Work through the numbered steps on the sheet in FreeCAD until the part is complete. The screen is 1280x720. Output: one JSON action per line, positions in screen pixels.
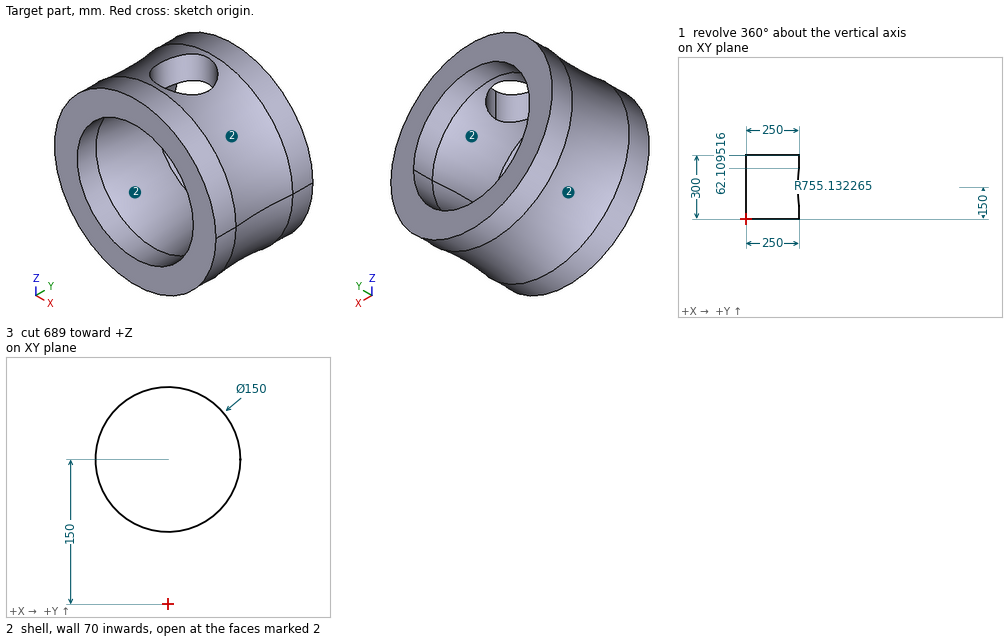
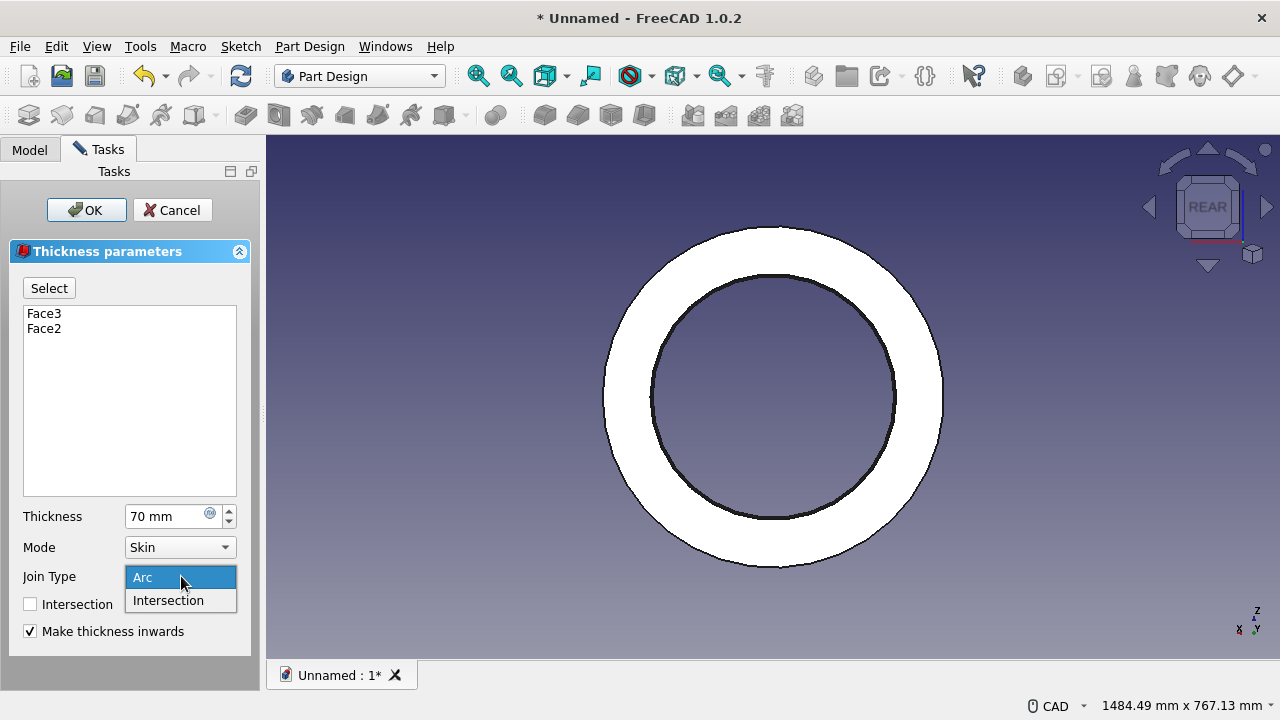
{"action": "left_click", "coordinate": [179, 600]}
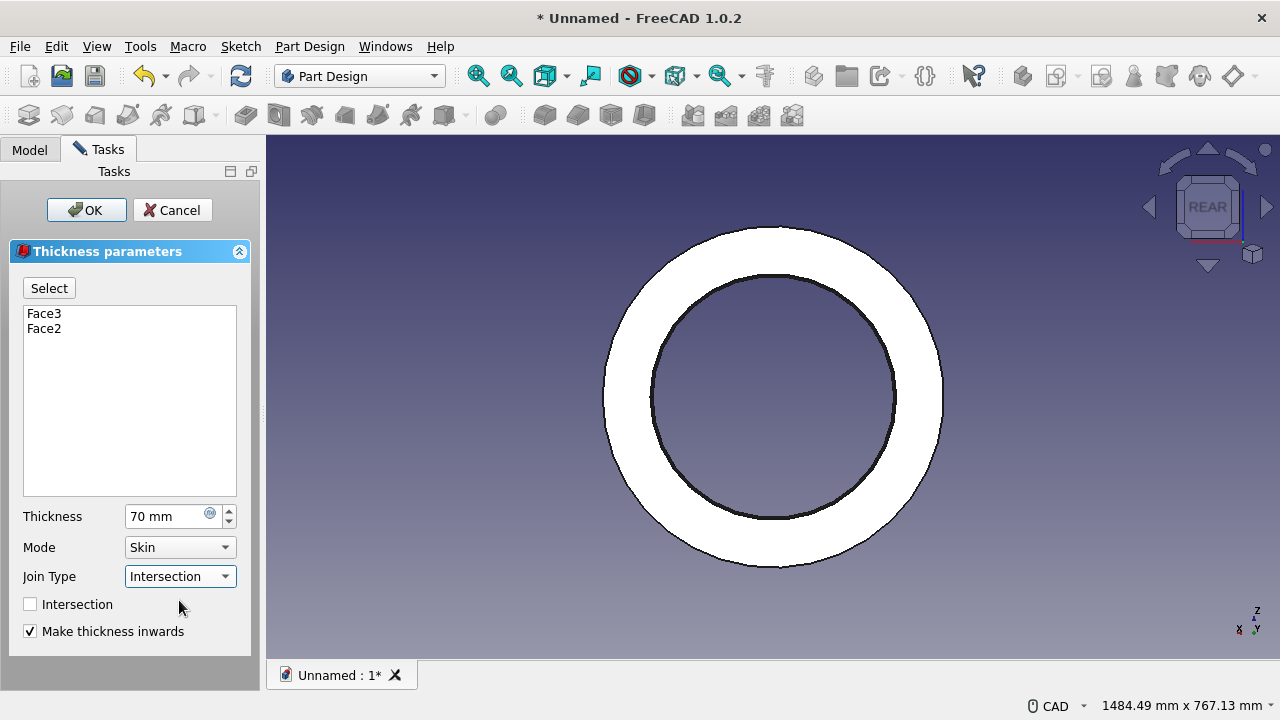
{"action": "left_click", "coordinate": [87, 210]}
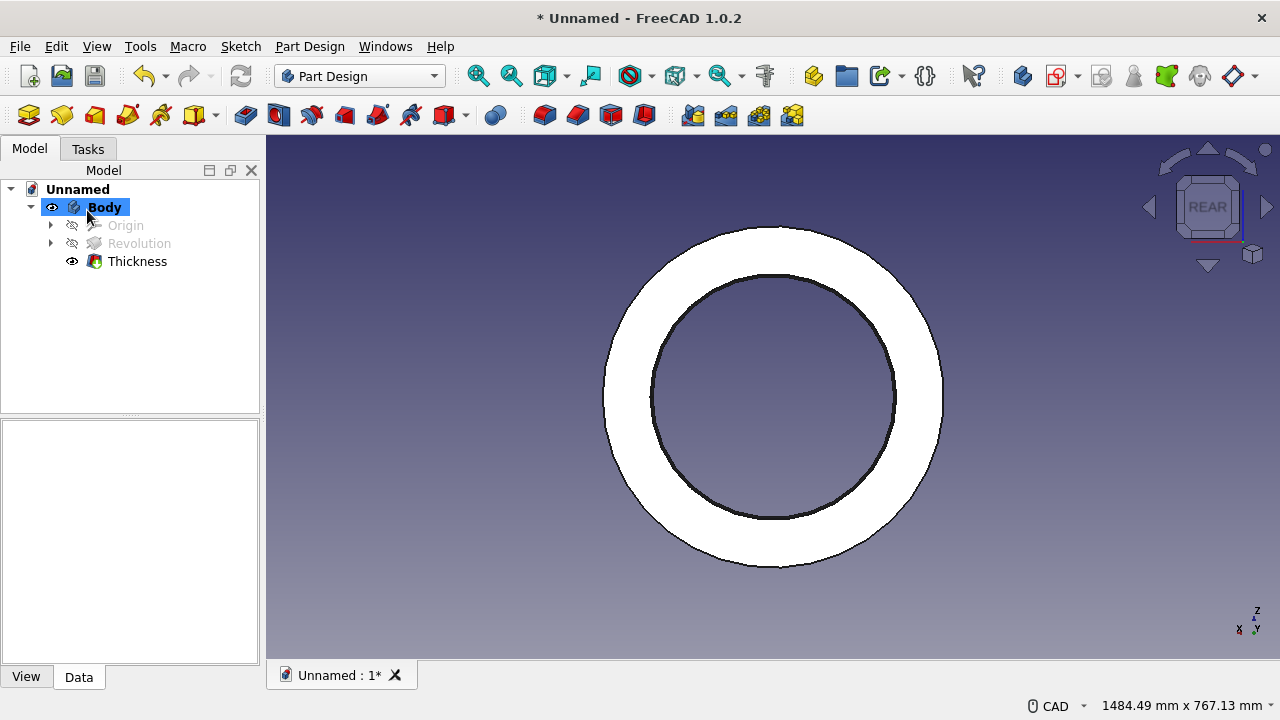
{"action": "left_click", "coordinate": [1056, 76]}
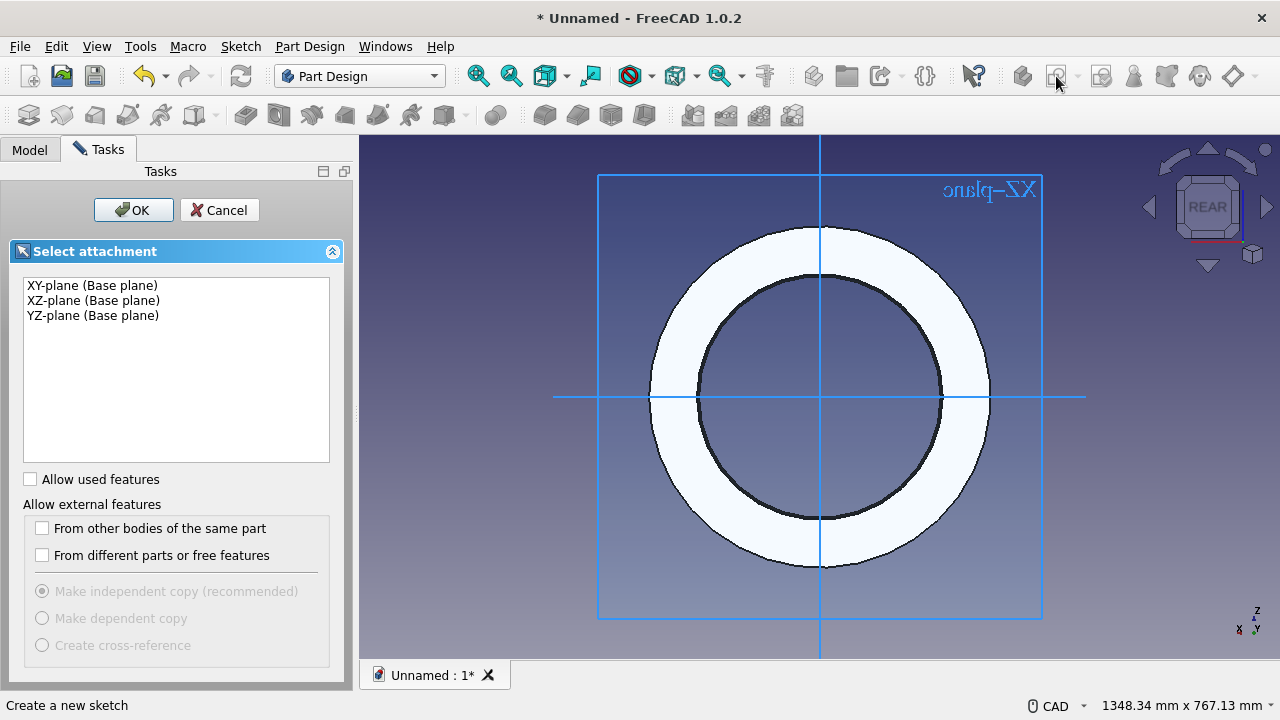
{"action": "left_click", "coordinate": [84, 286]}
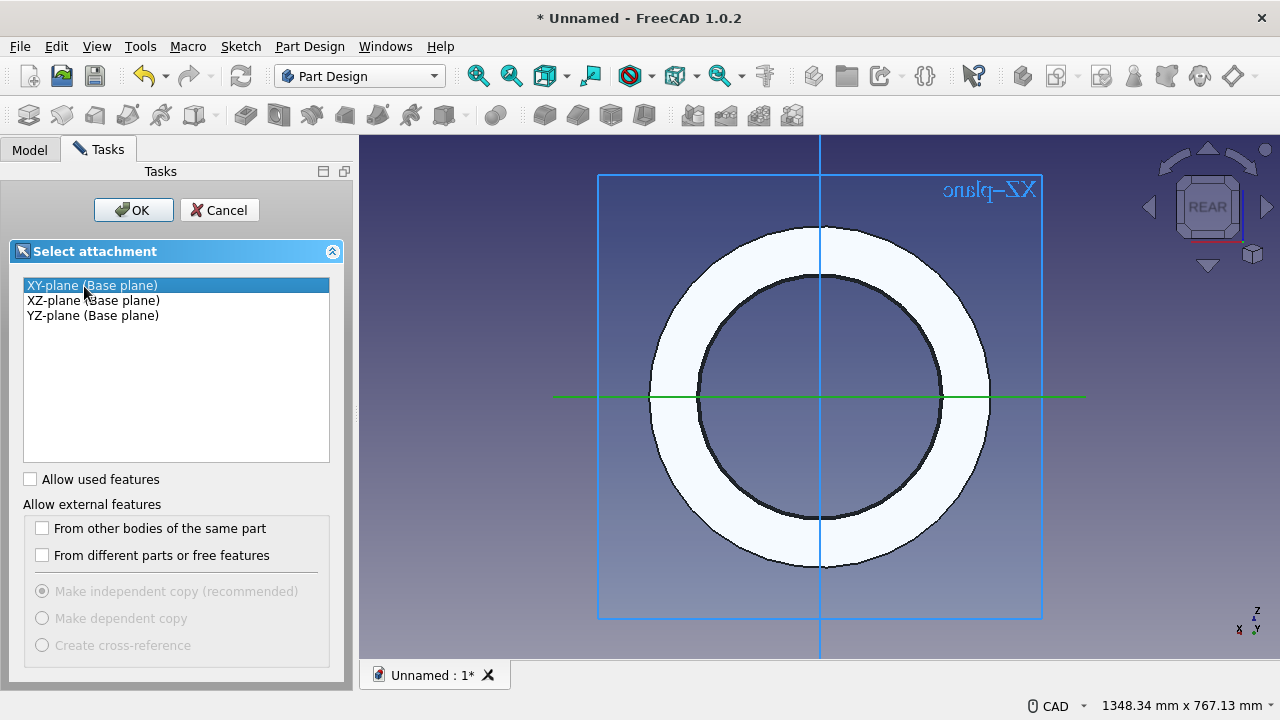
{"action": "left_click", "coordinate": [134, 210]}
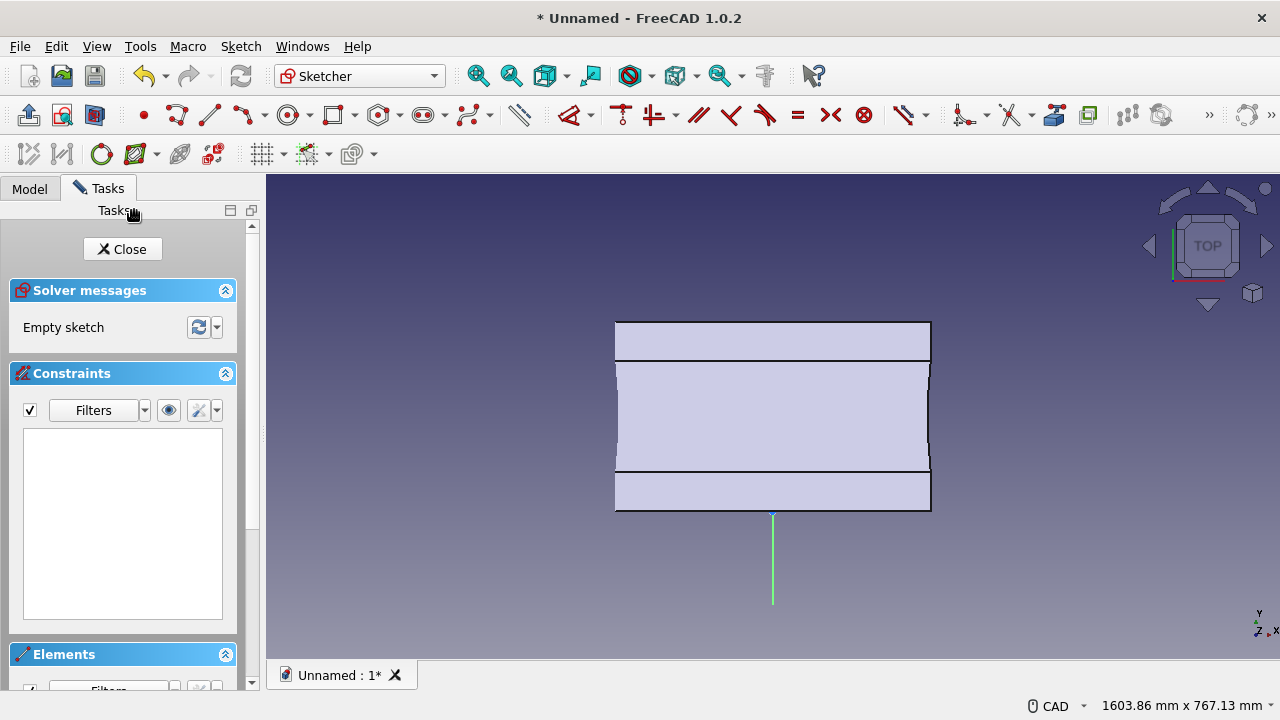
{"action": "left_click", "coordinate": [95, 116]}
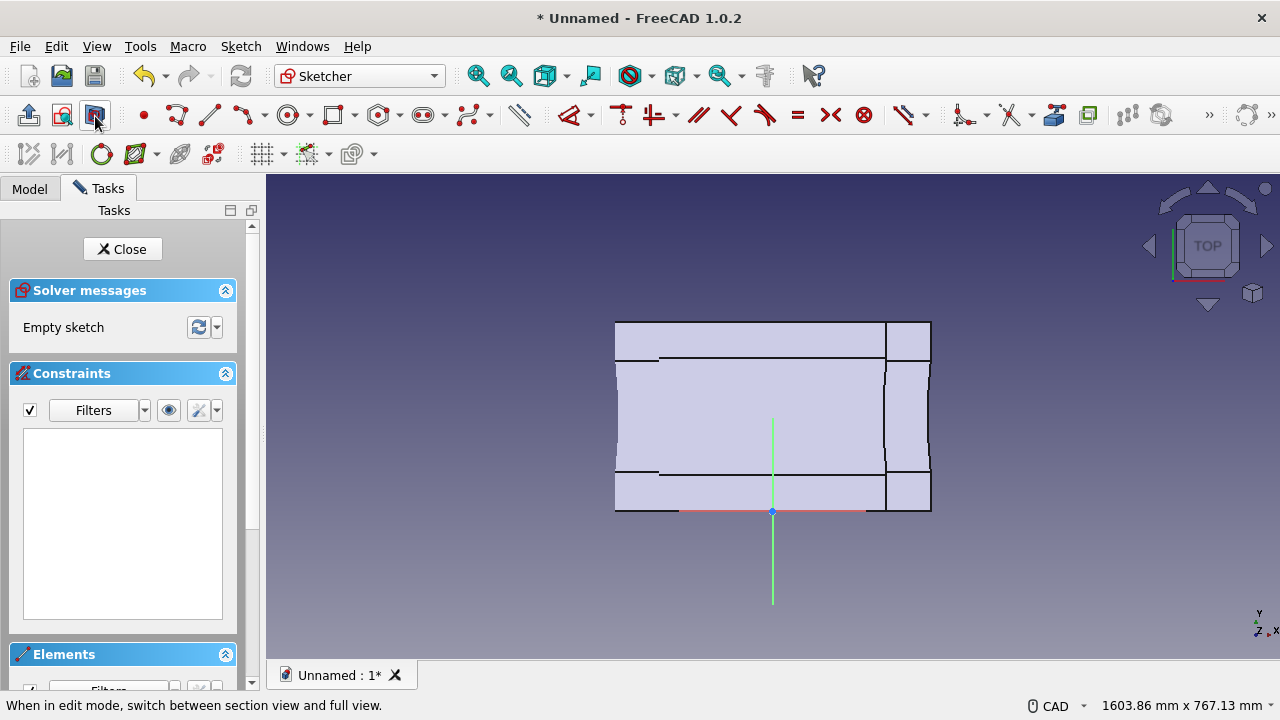
{"action": "scroll", "coordinate": [828, 460], "scroll_direction": "up", "scroll_amount": 4}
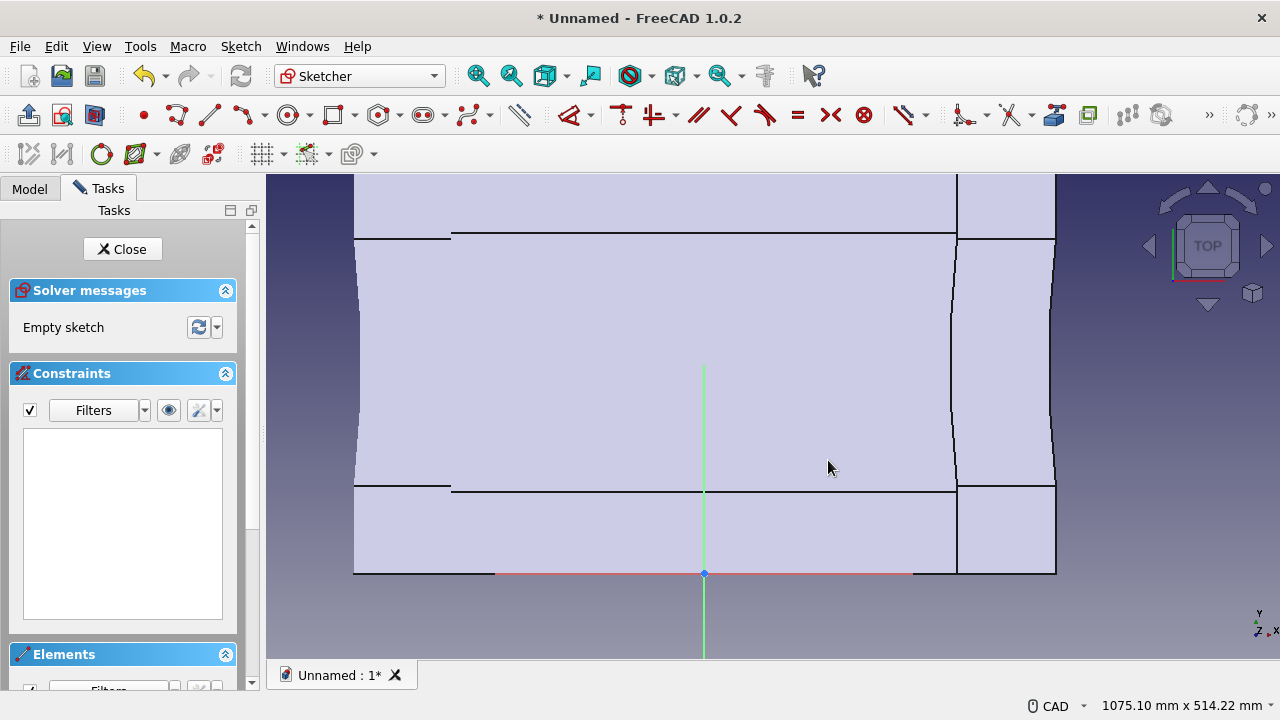
{"action": "left_click", "coordinate": [288, 116]}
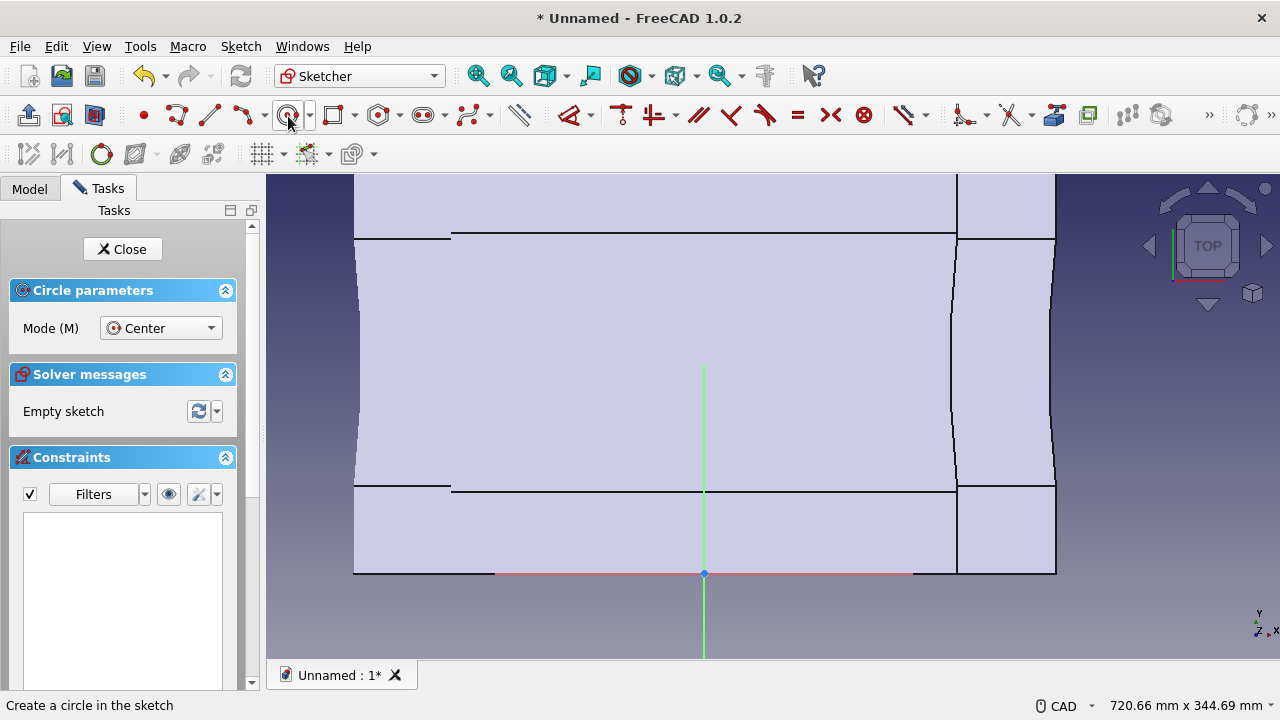
{"action": "left_click", "coordinate": [704, 362]}
{"action": "mouse_move", "coordinate": [779, 288]}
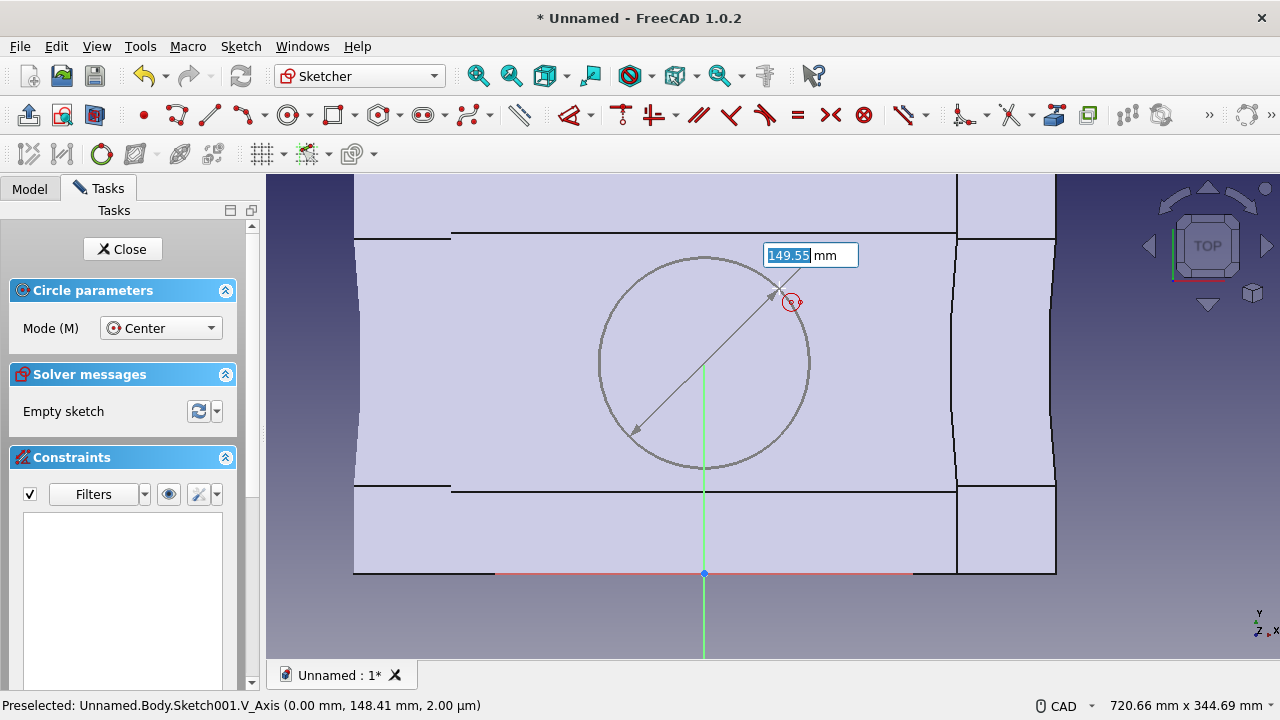
{"action": "type", "text": "150"}
{"action": "key", "text": "Return"}
{"action": "key", "text": "Escape"}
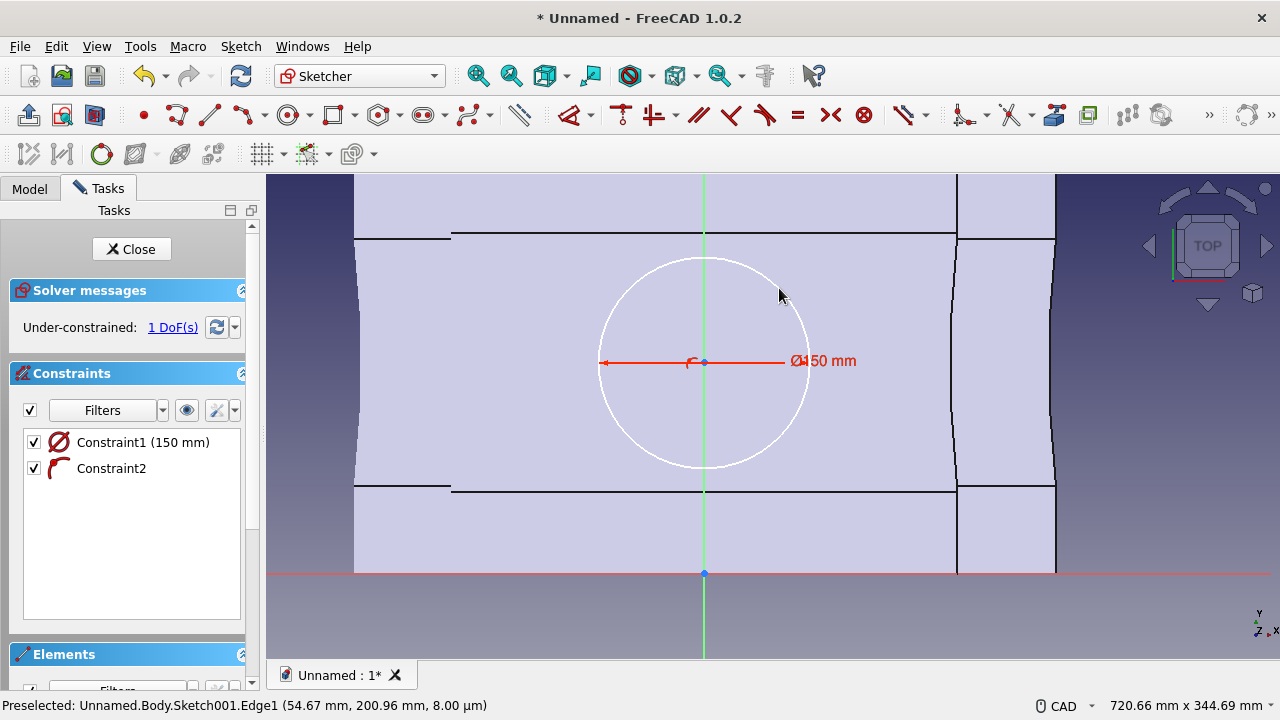
{"action": "left_click", "coordinate": [568, 116]}